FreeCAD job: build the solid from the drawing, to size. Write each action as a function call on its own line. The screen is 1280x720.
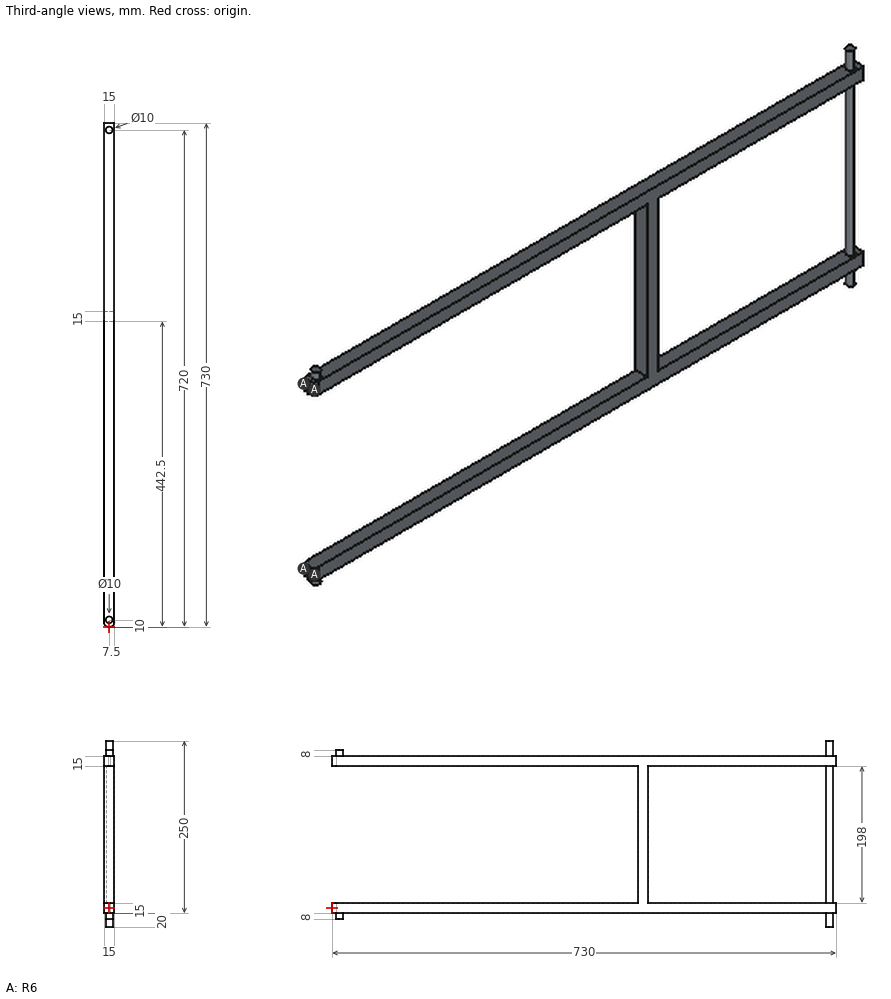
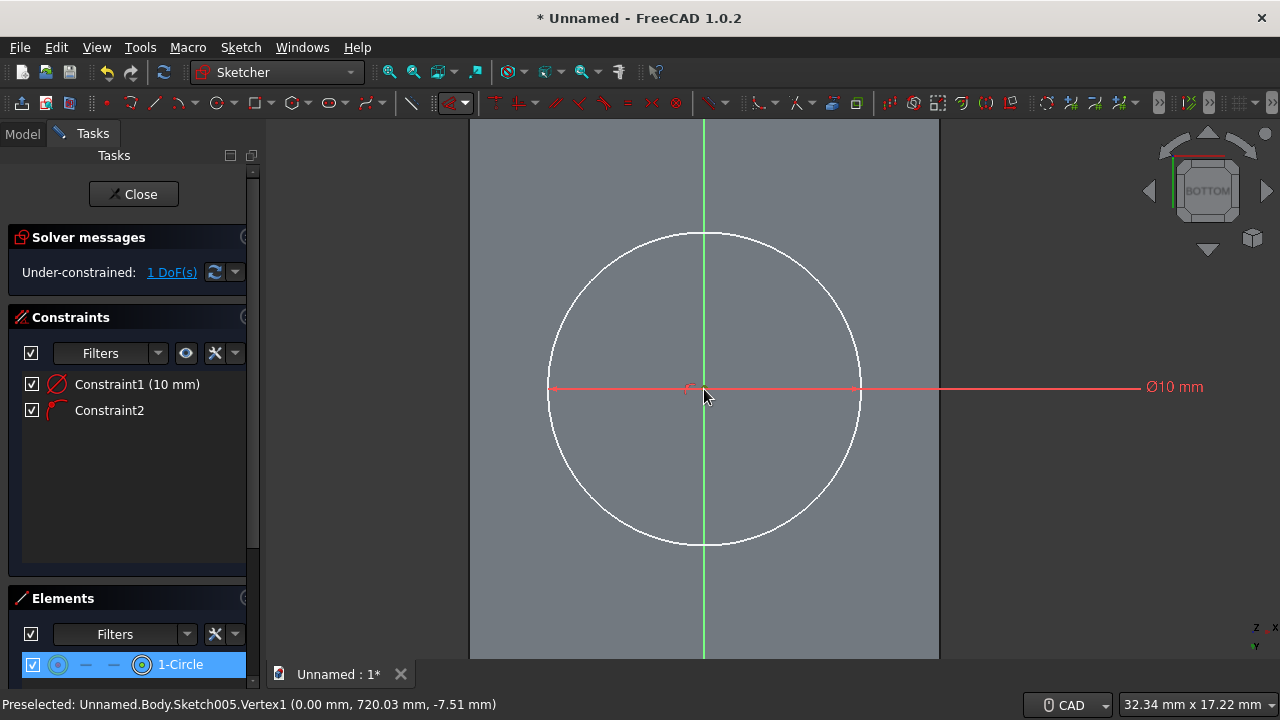
key(i)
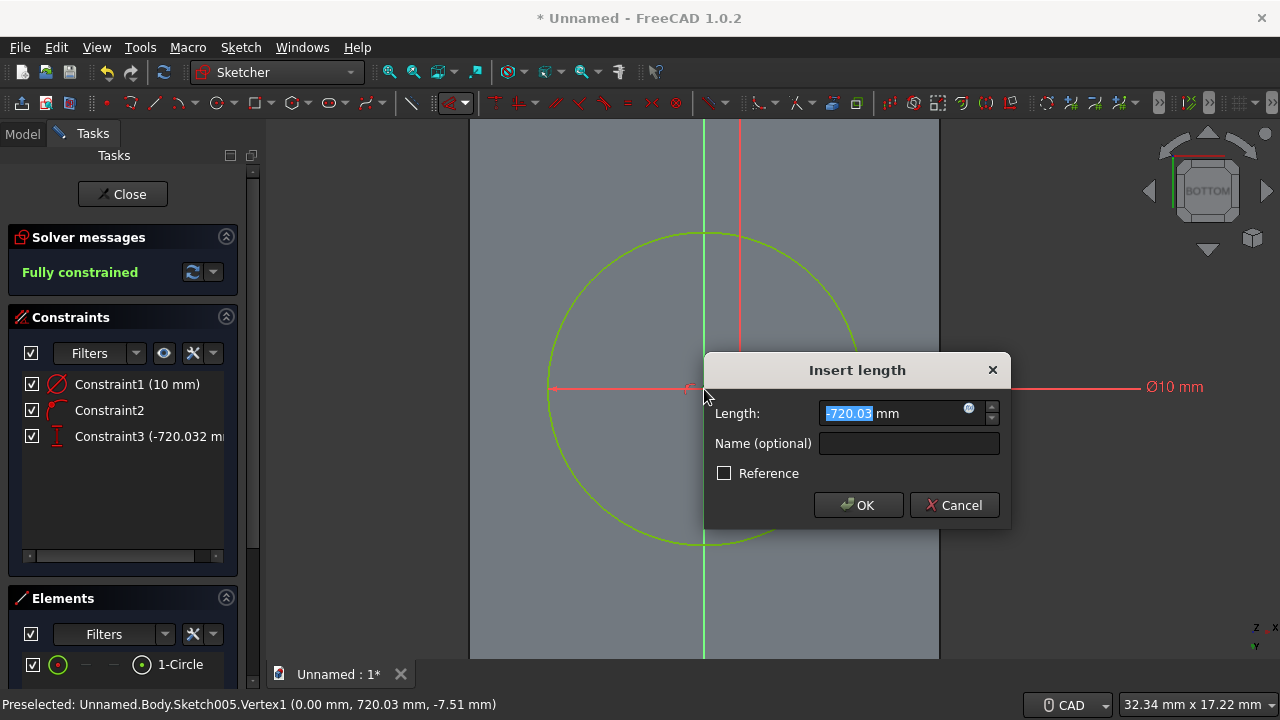
text(-720)
key(Return)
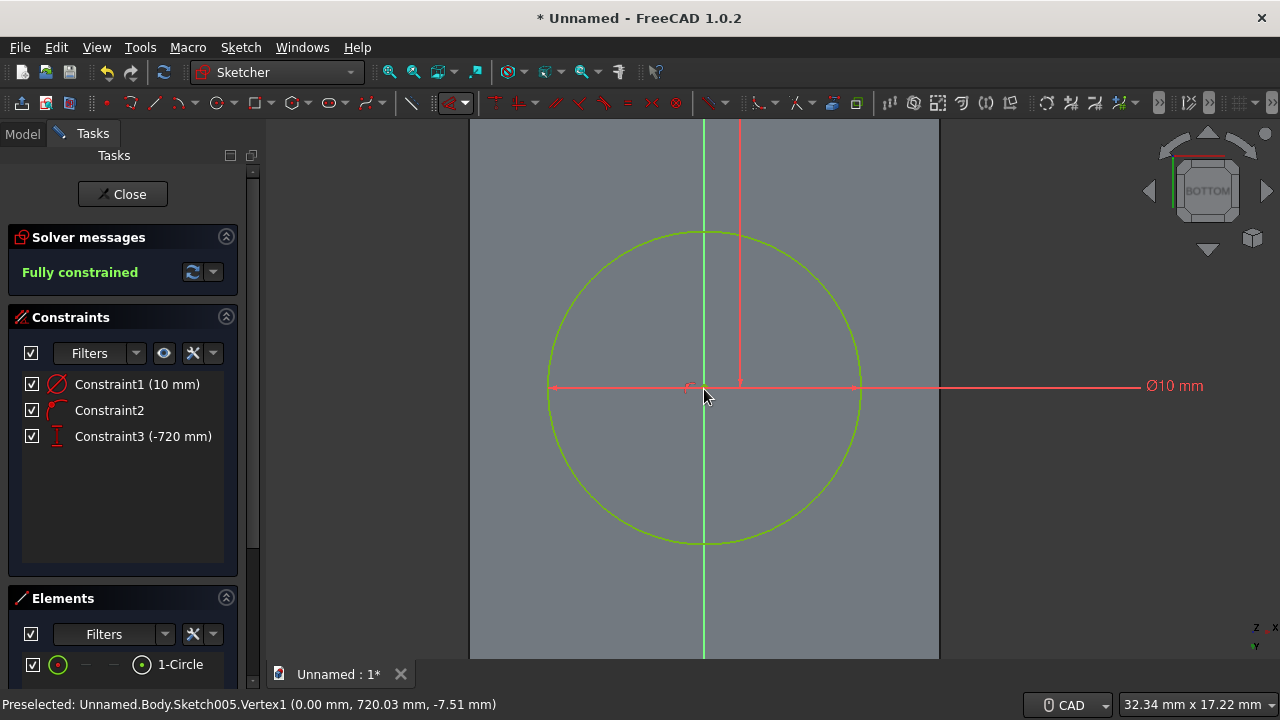
click(123, 194)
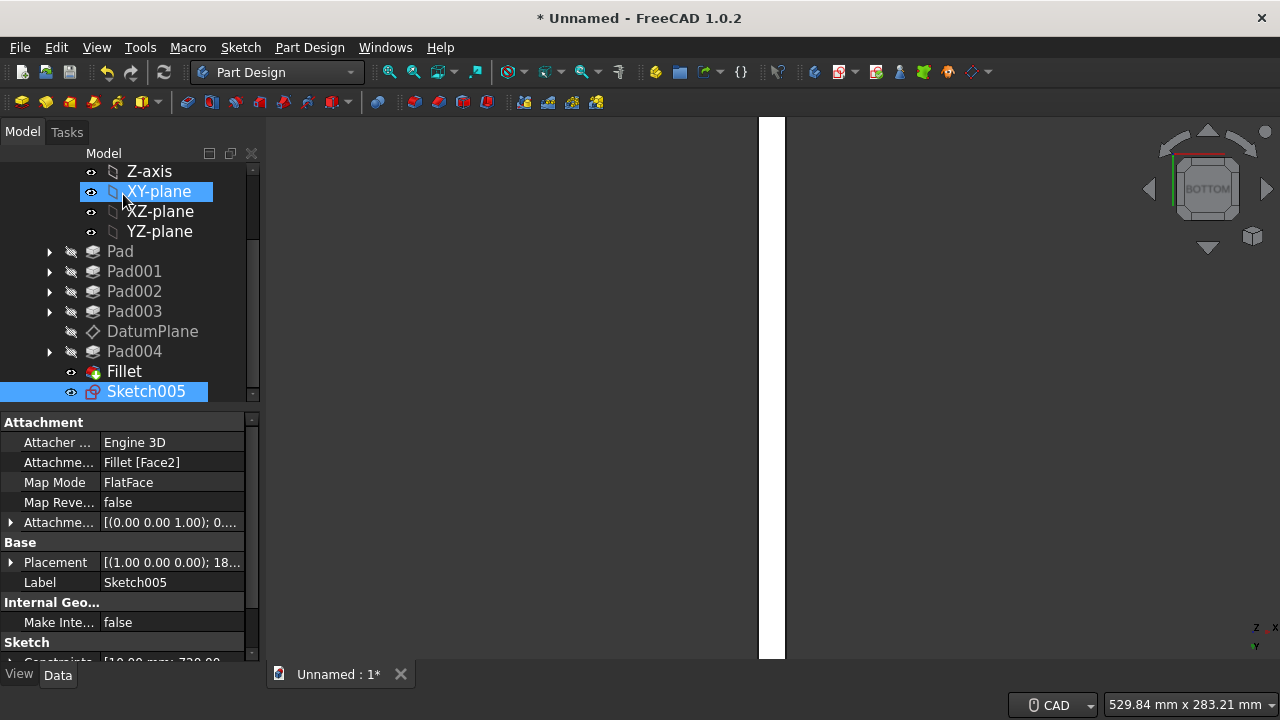
click(22, 102)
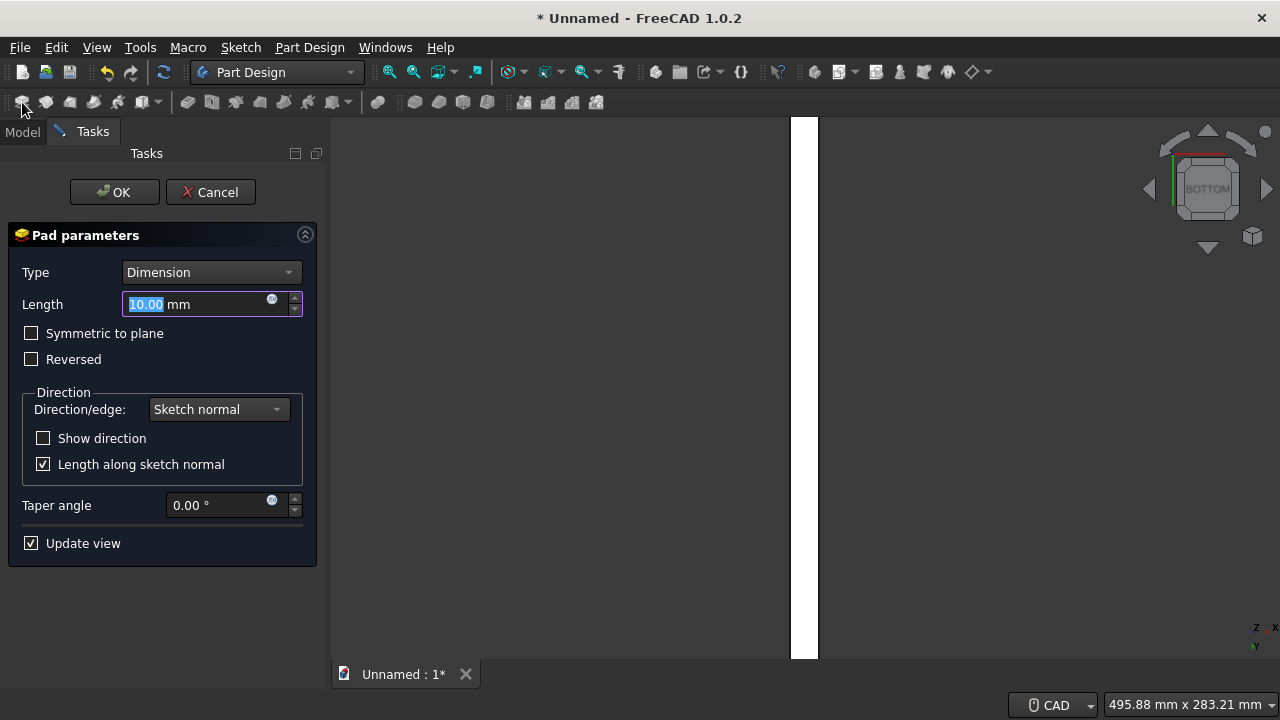
click(212, 272)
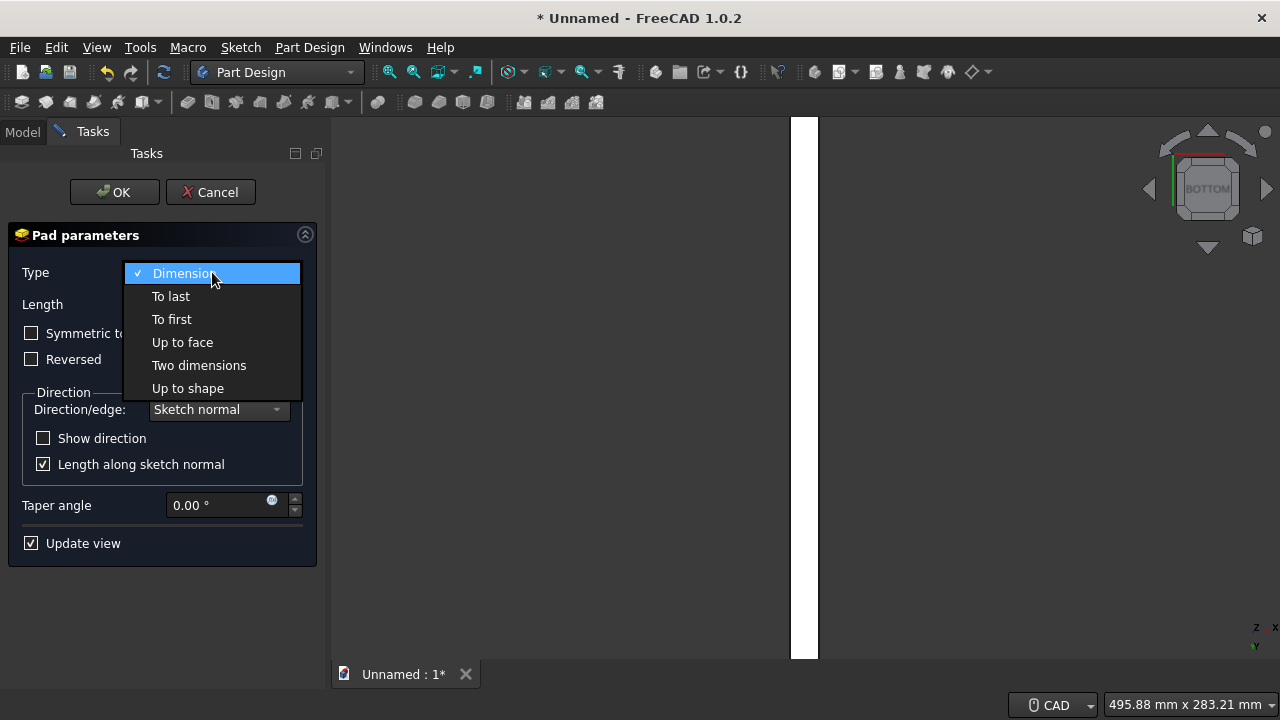
click(212, 366)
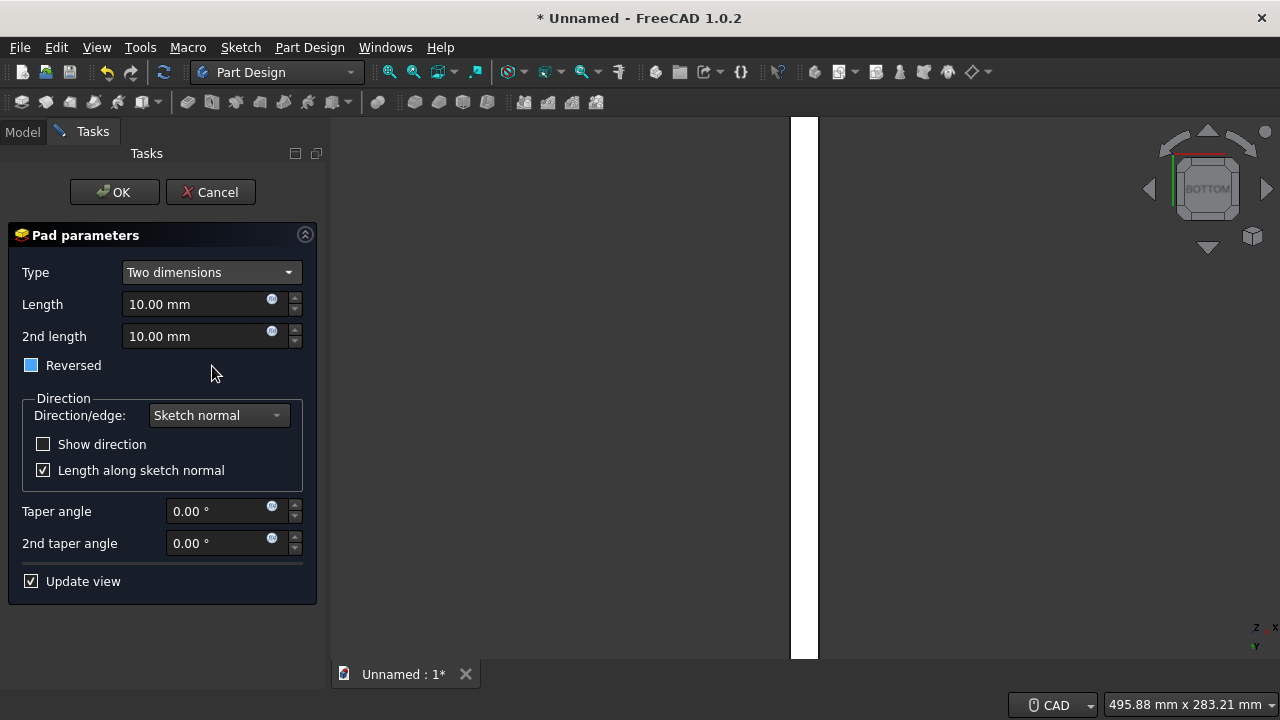
triple_click(204, 304)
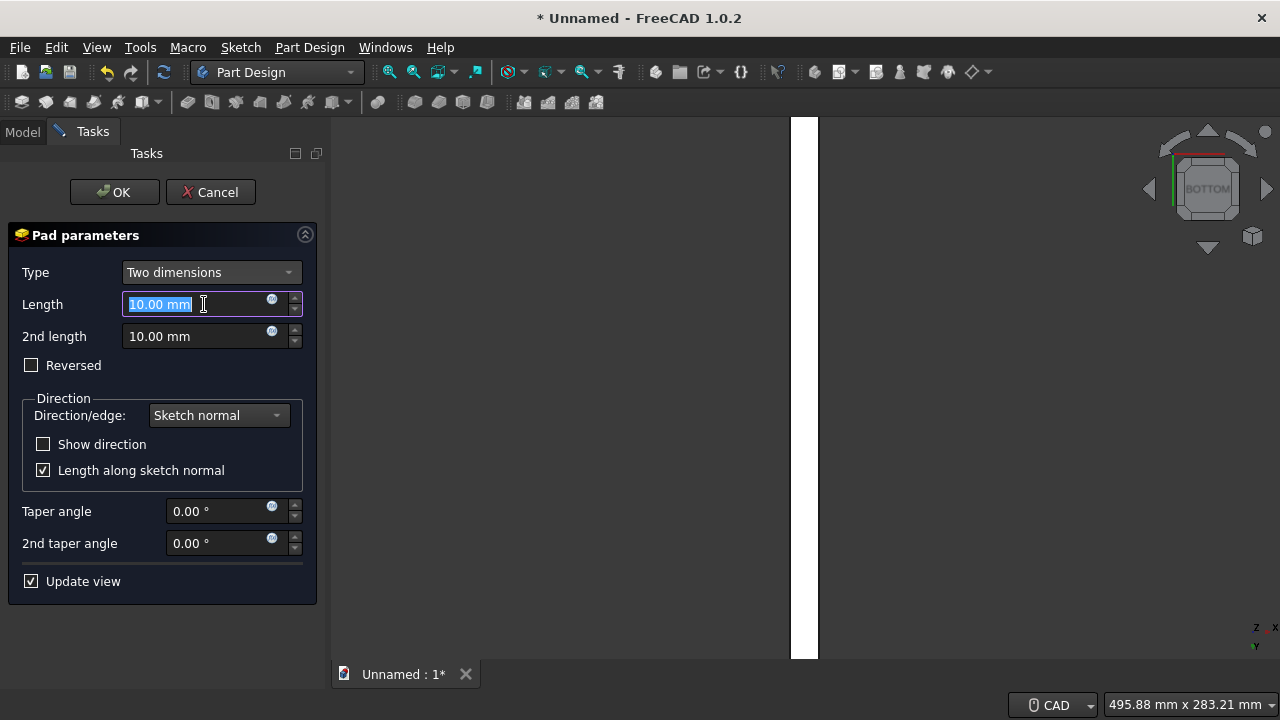
text(20)
key(Tab)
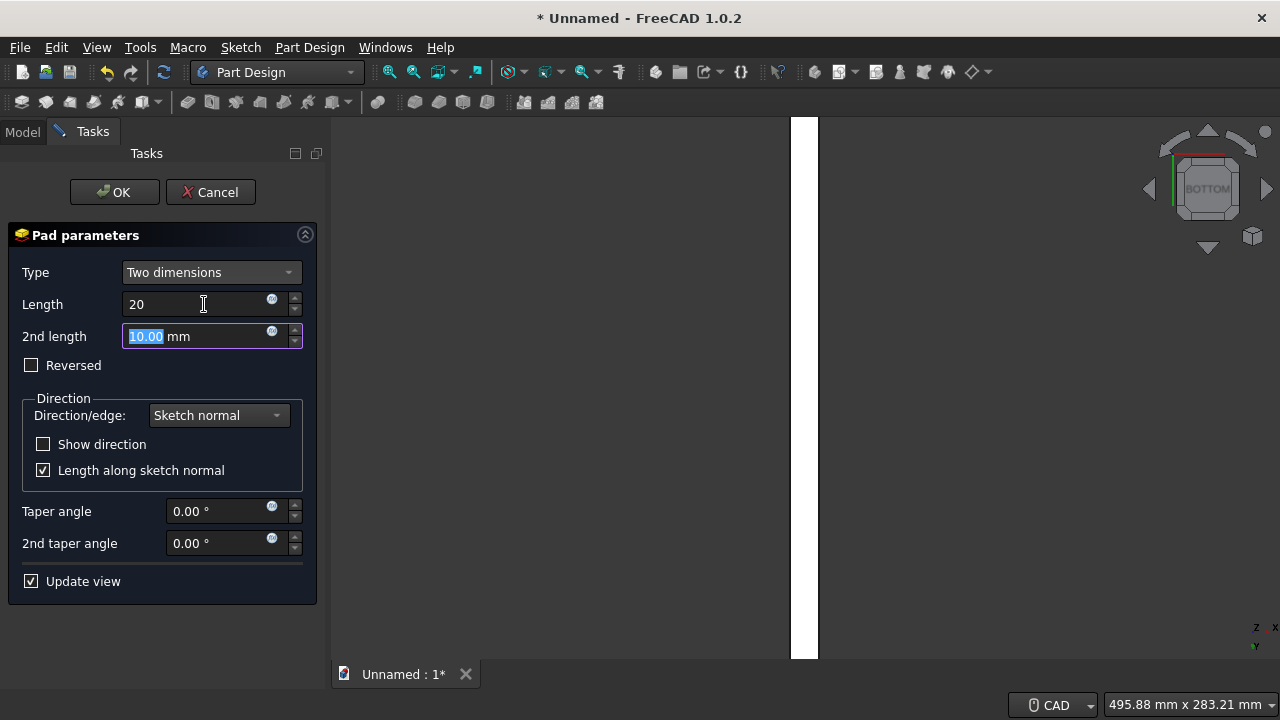
text(250)
key(Tab)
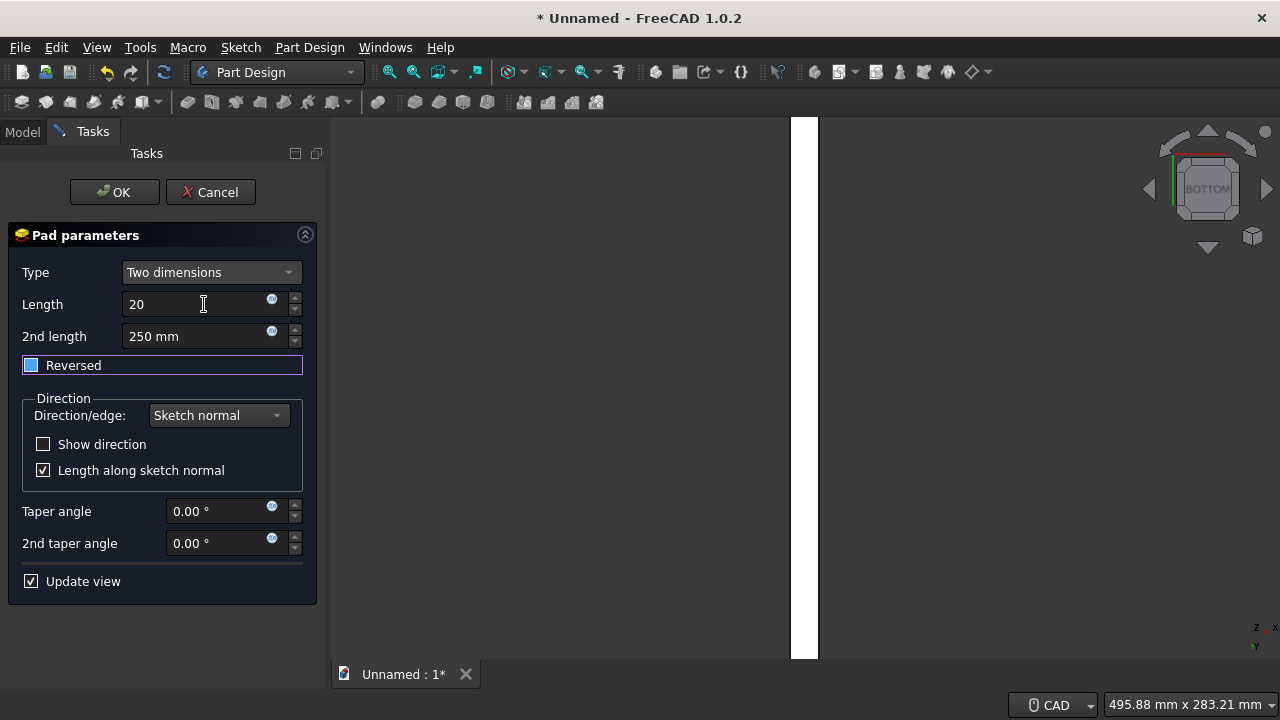
click(115, 192)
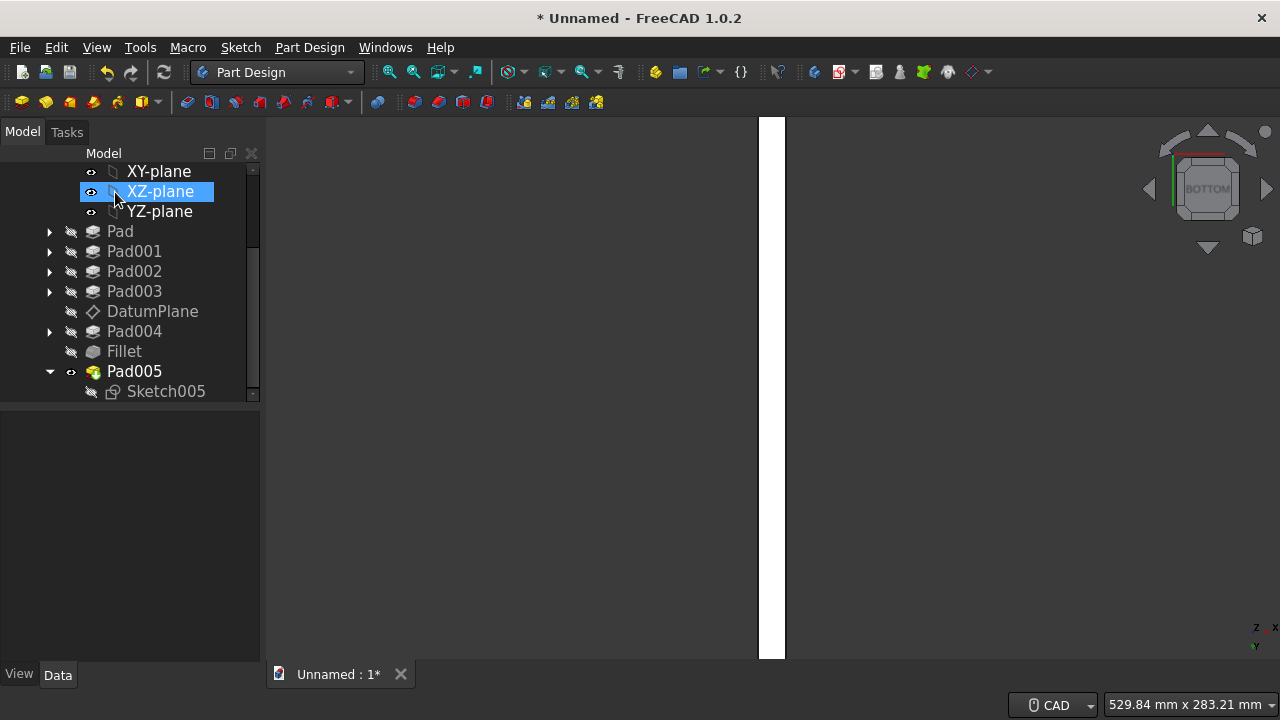
key(0)